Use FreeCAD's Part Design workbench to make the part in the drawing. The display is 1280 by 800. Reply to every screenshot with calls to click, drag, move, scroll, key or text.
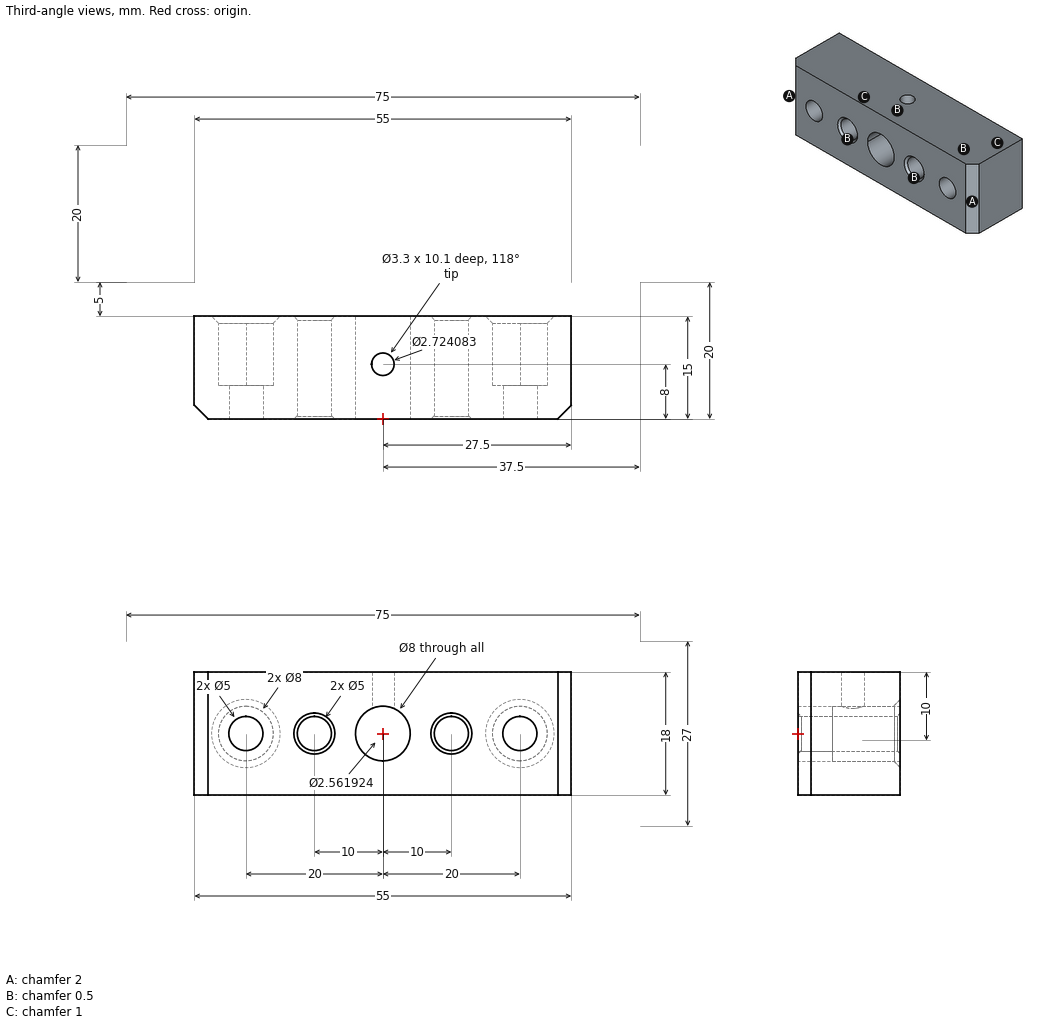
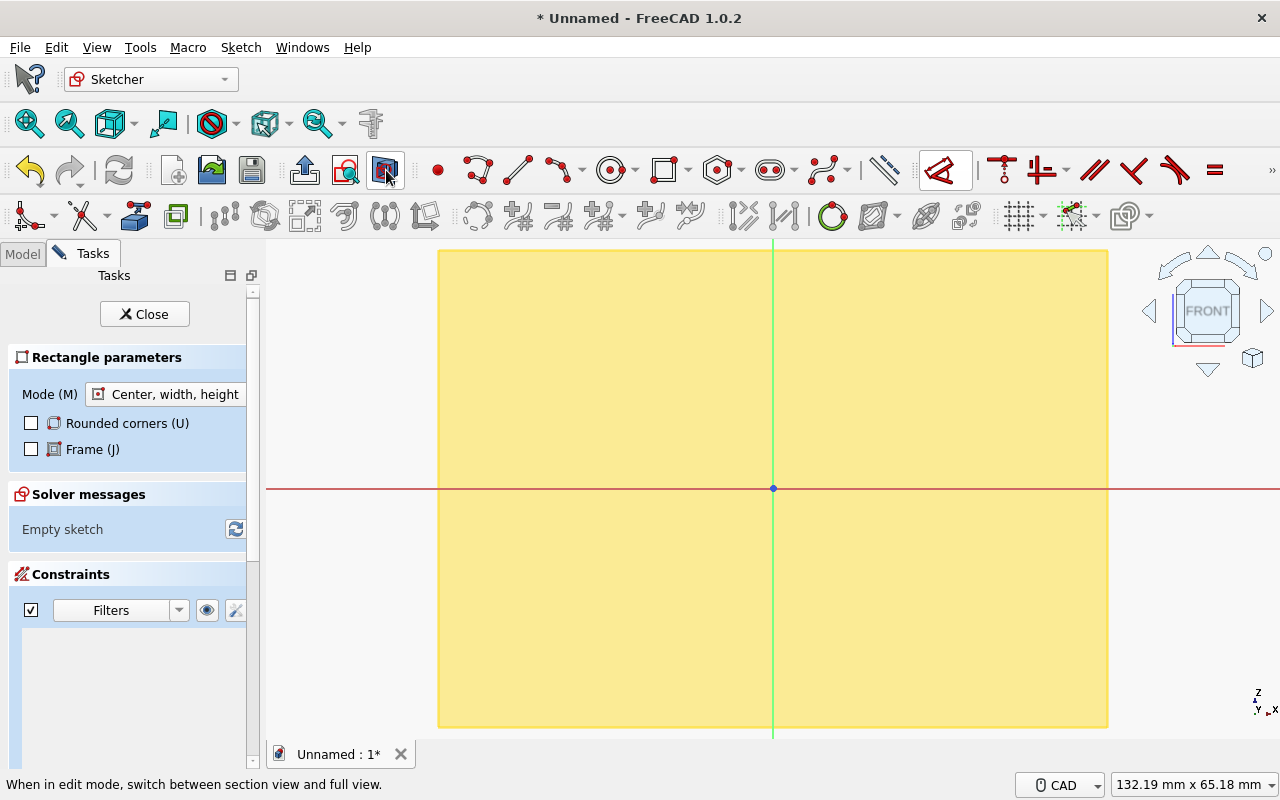
click(773, 489)
move(1061, 420)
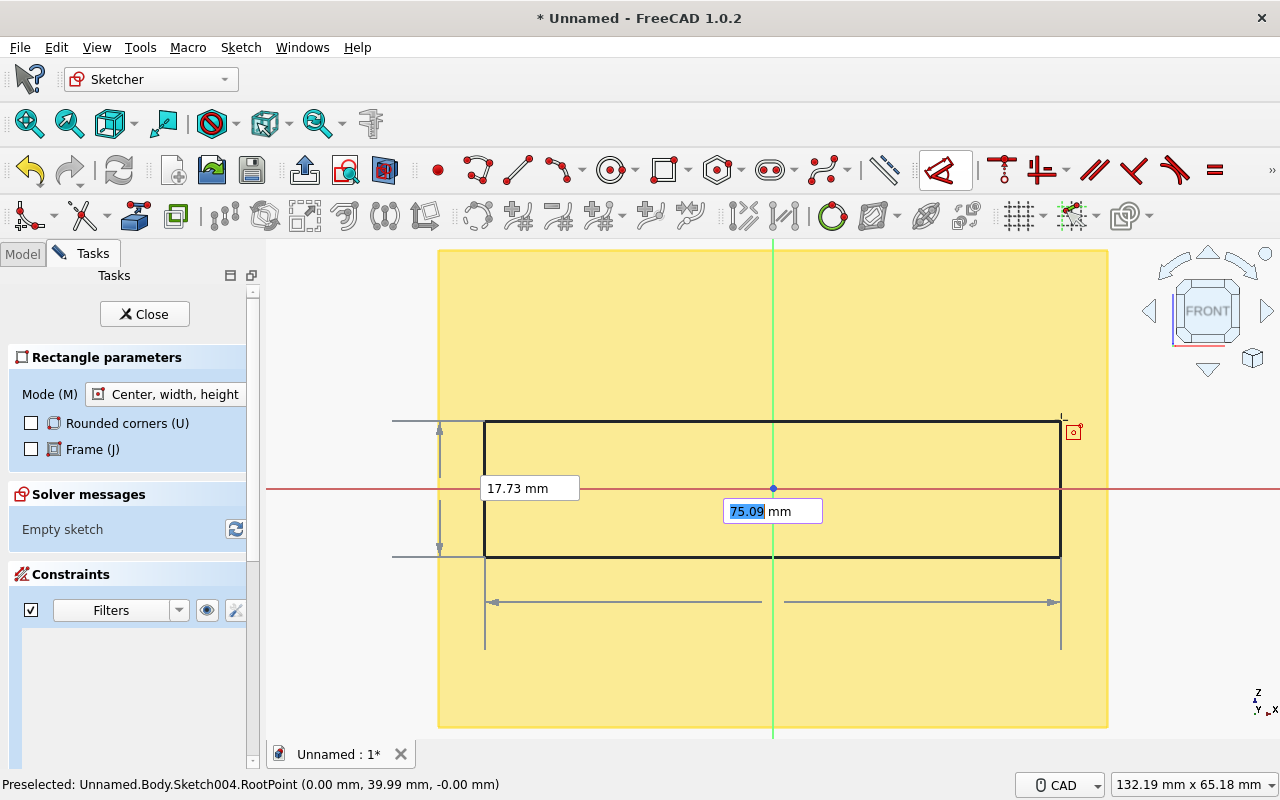
text(75)
key(Tab)
text(18)
key(Return)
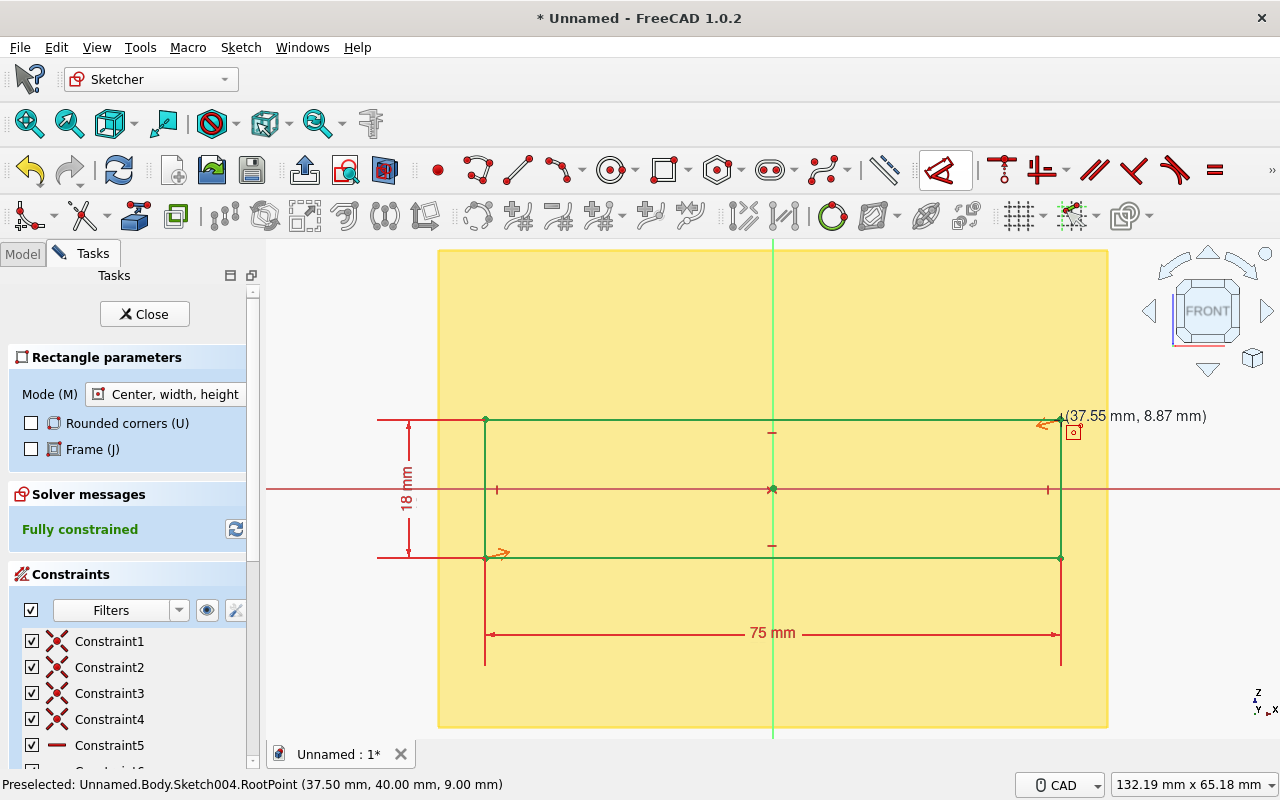
click(612, 170)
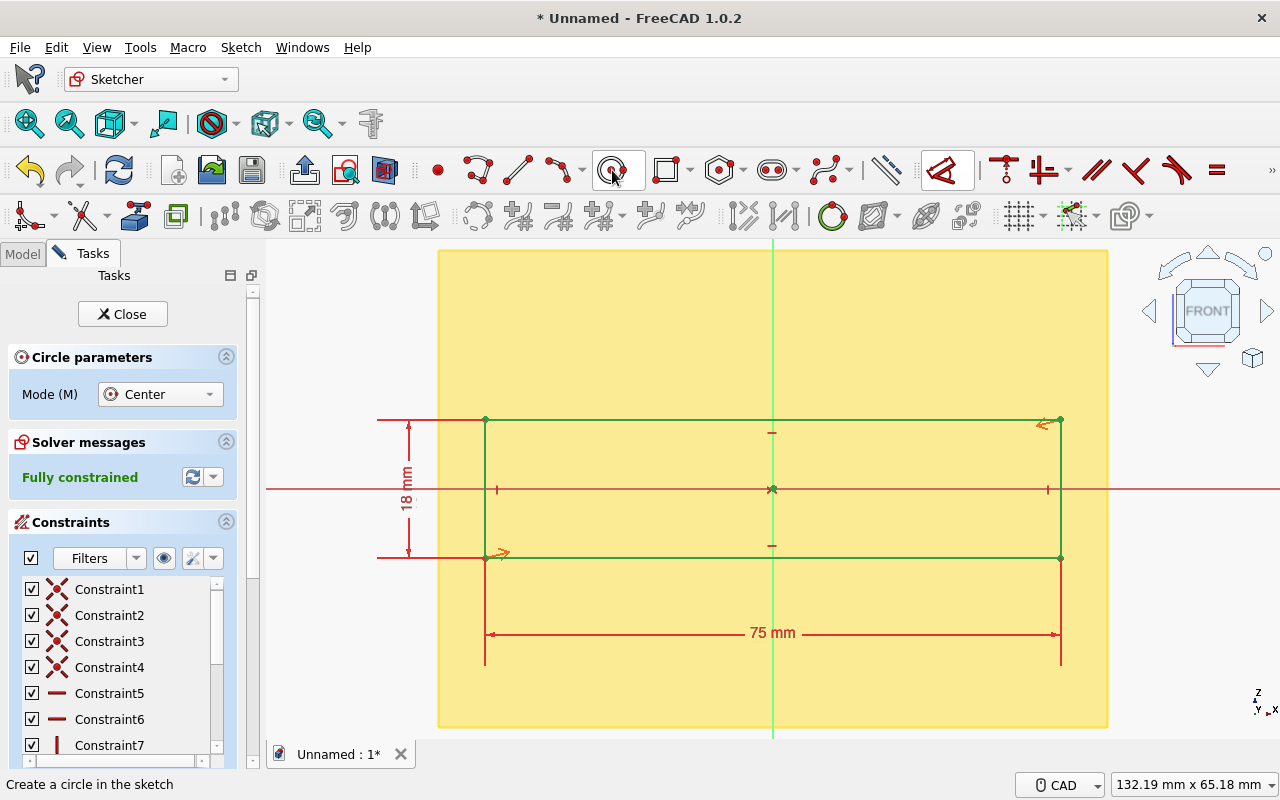
click(620, 489)
move(641, 467)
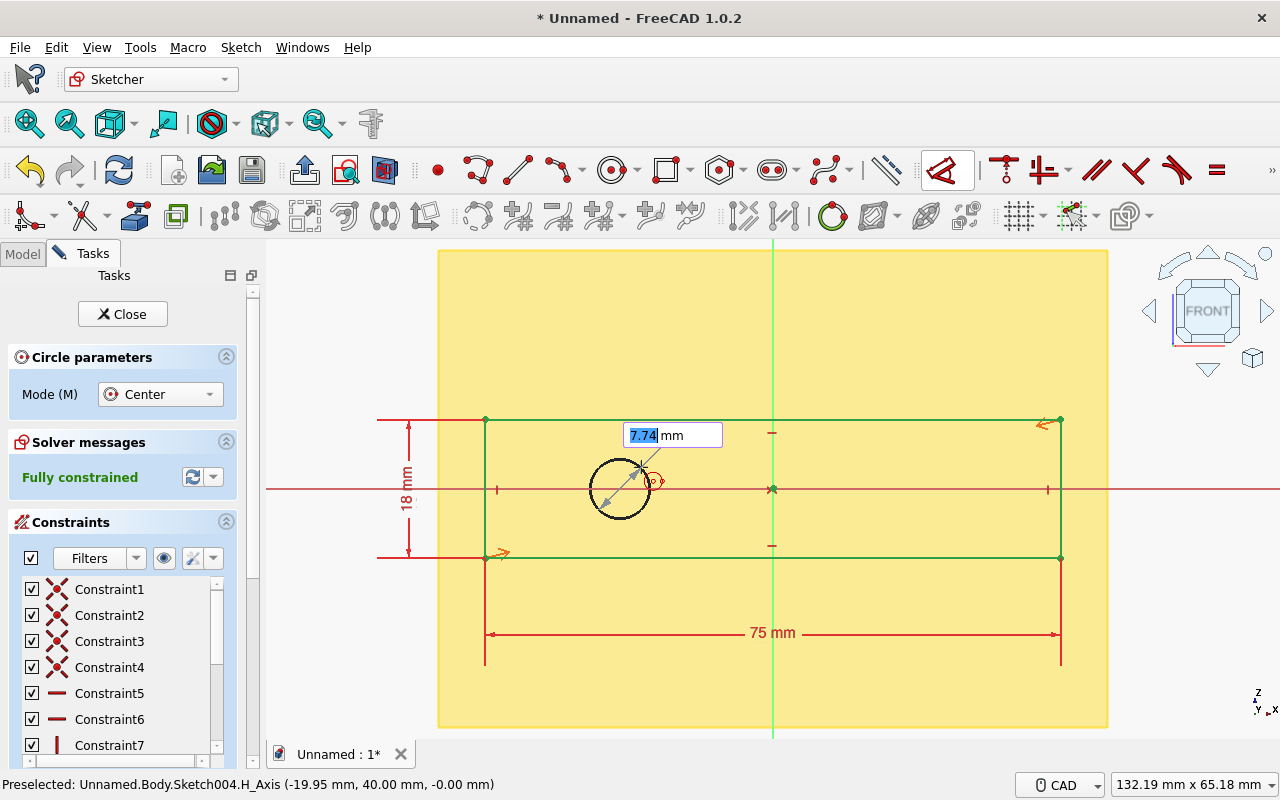
text(8)
key(Return)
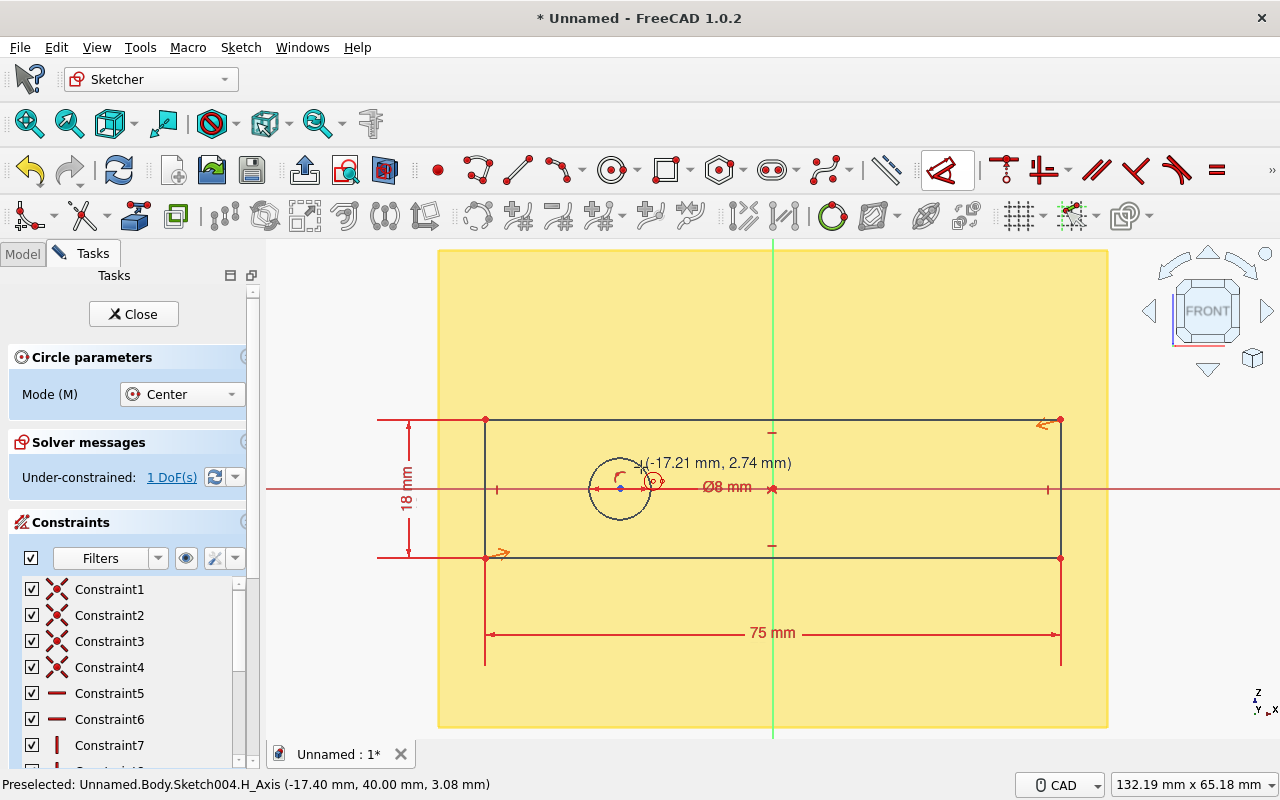
click(926, 489)
move(948, 467)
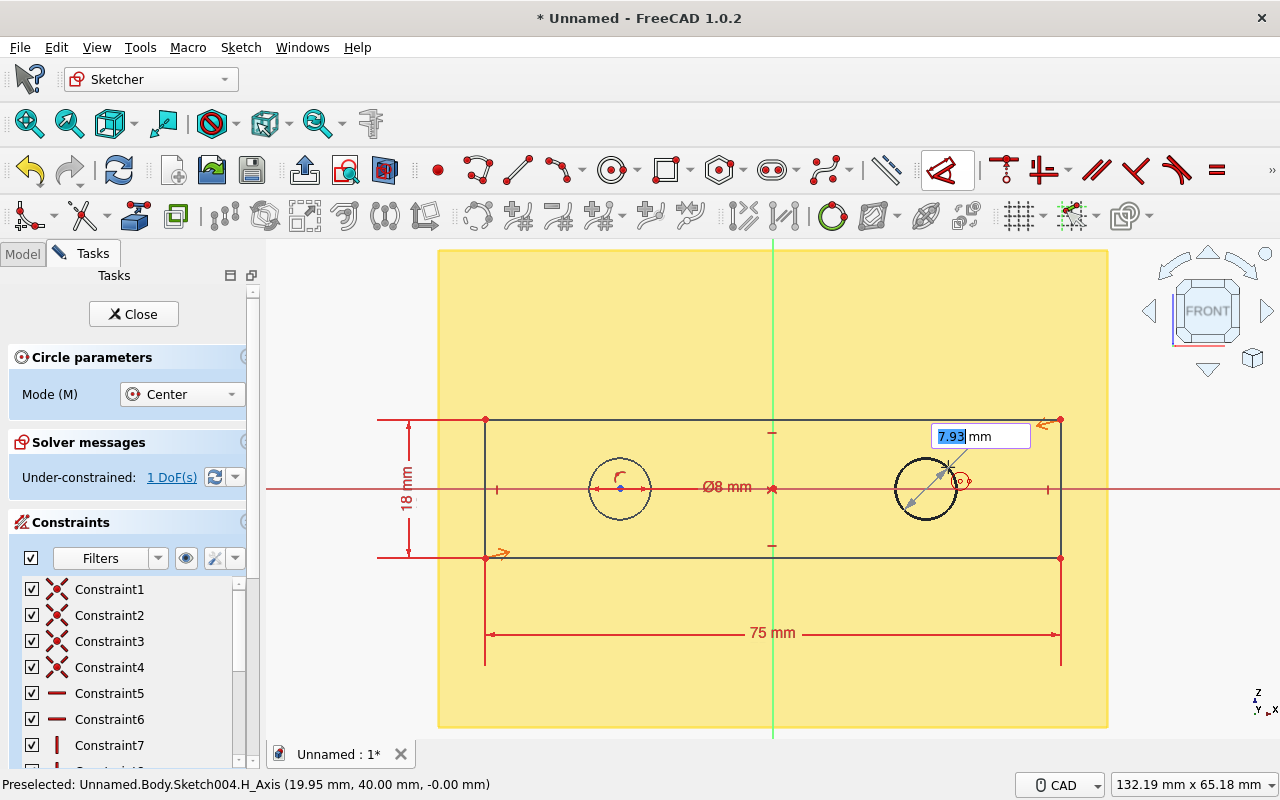
text(8)
key(Return)
key(Escape)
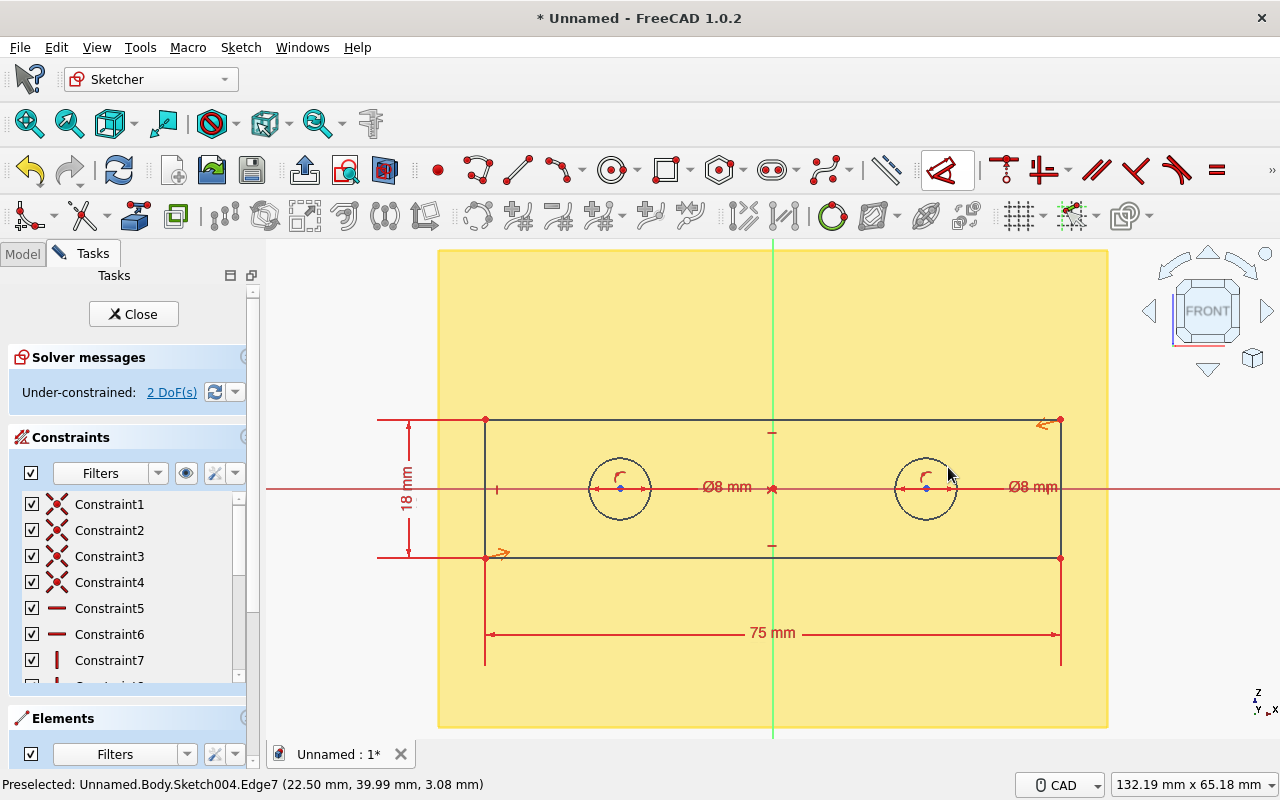
click(620, 489)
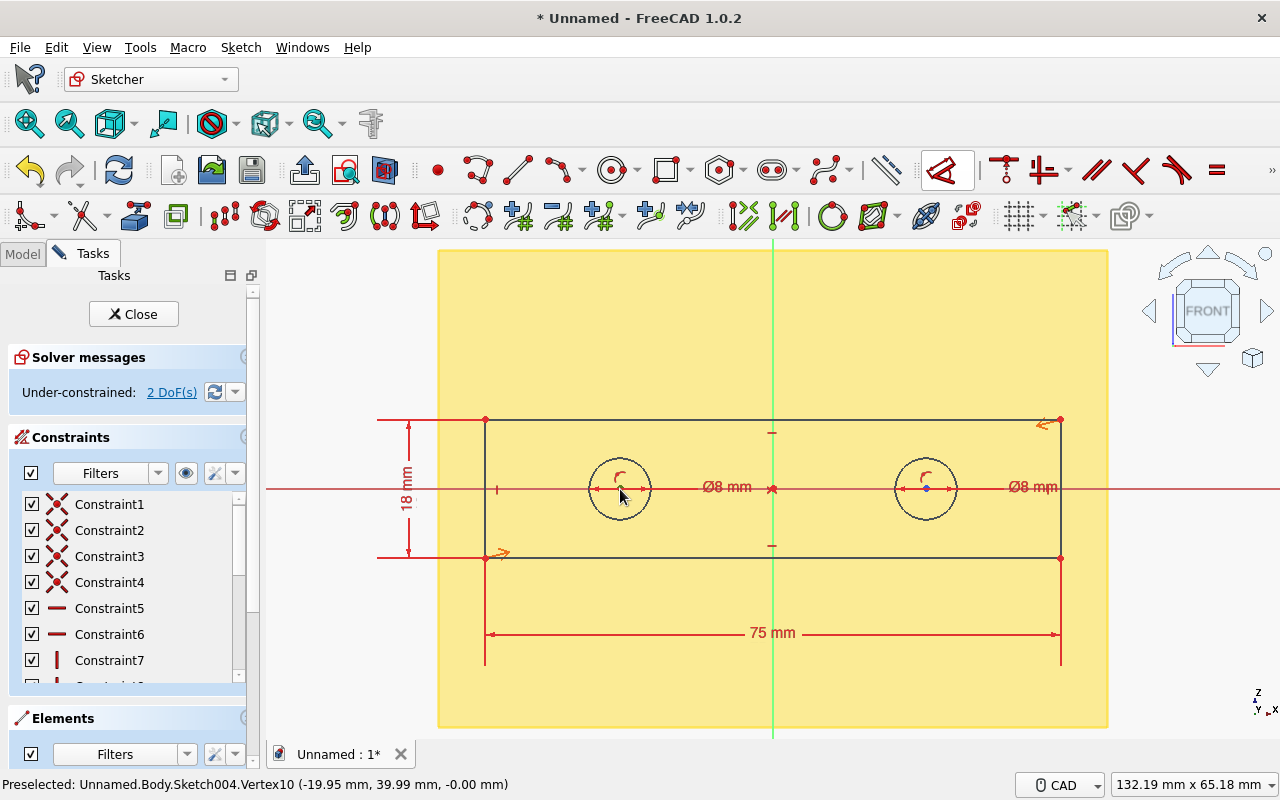
key(l)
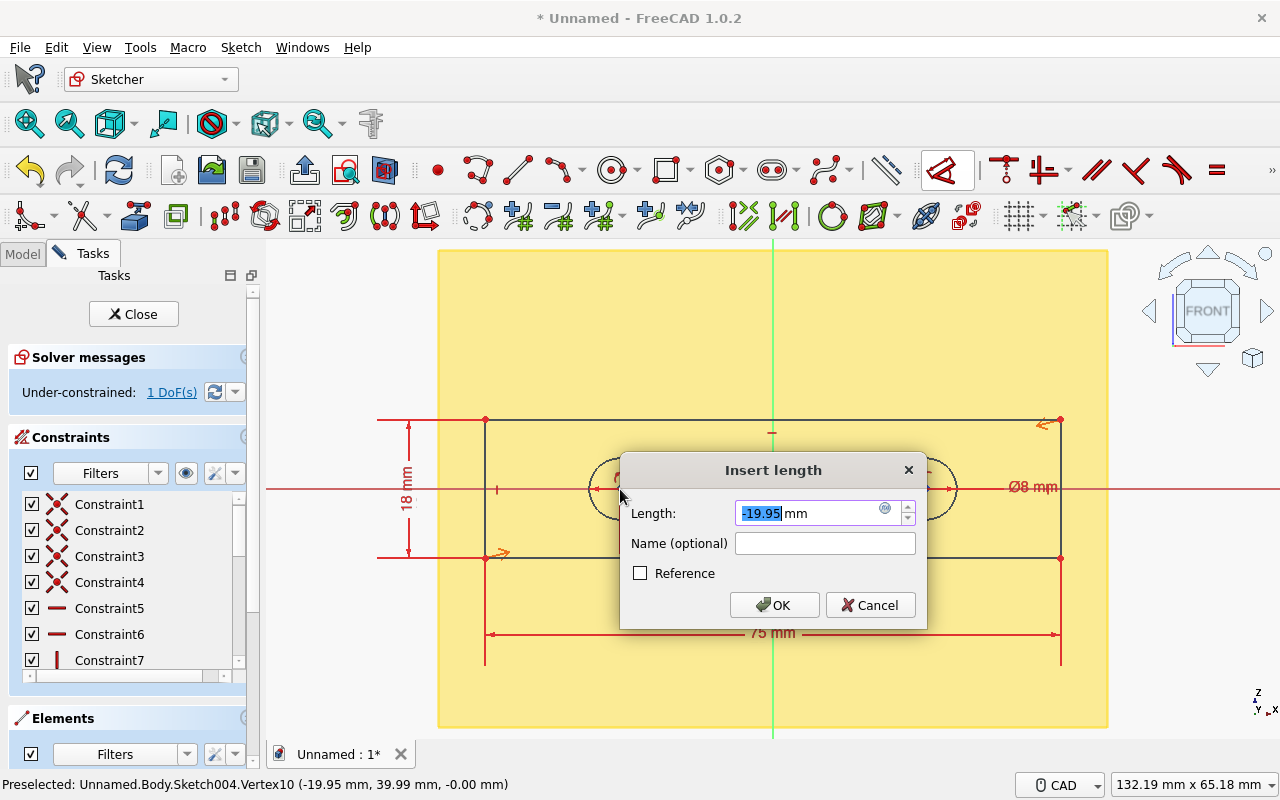
text(-20)
key(Return)